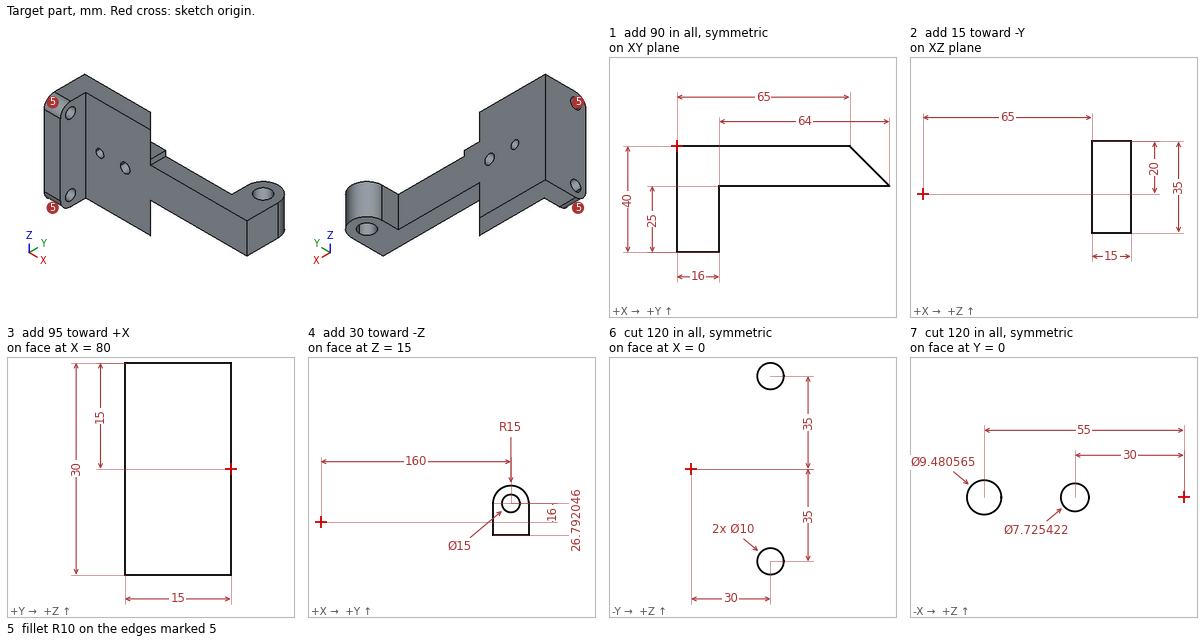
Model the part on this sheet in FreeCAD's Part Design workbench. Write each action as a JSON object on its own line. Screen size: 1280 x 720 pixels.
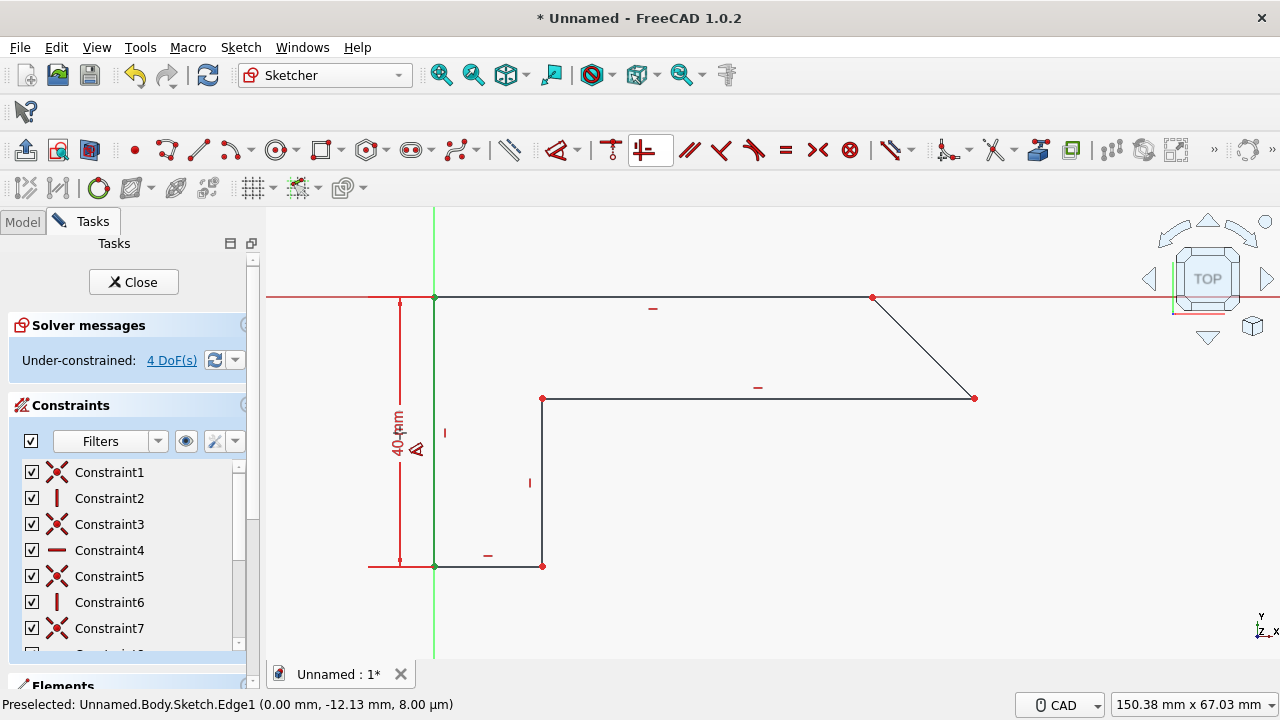
{"action": "left_click", "coordinate": [467, 567]}
{"action": "left_click", "coordinate": [488, 601]}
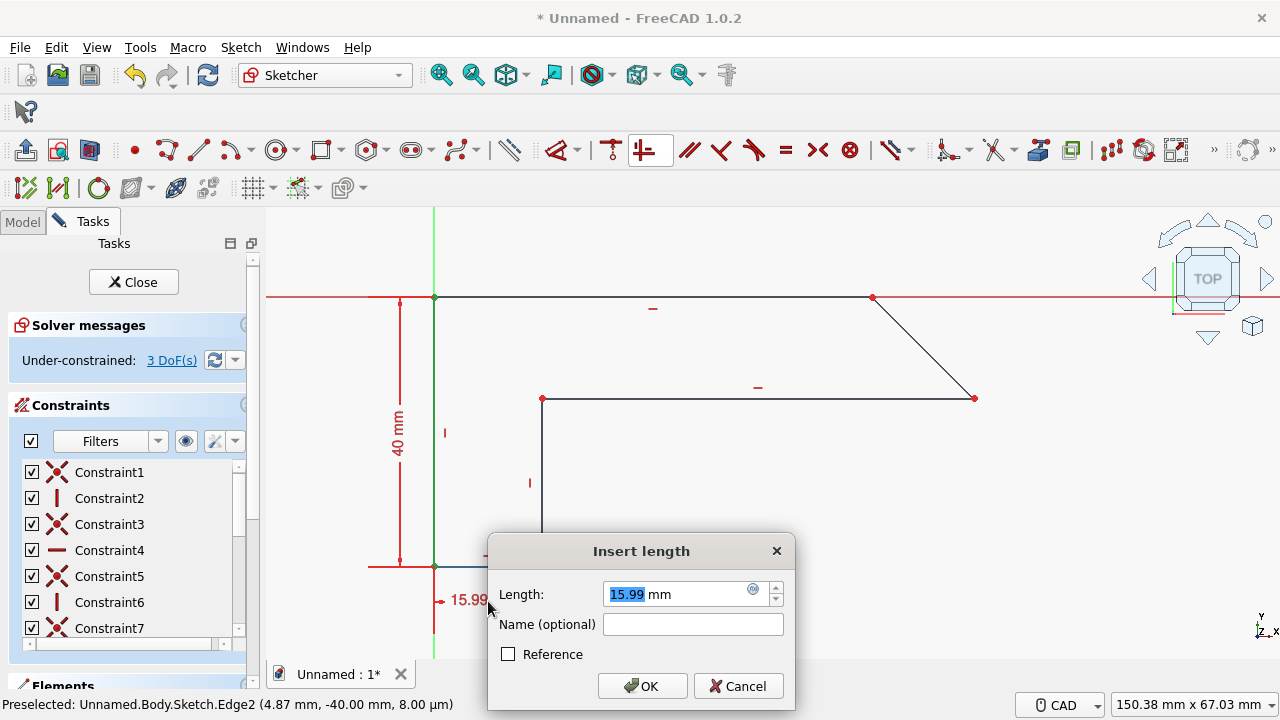
{"action": "type", "text": "16"}
{"action": "key", "text": "Return"}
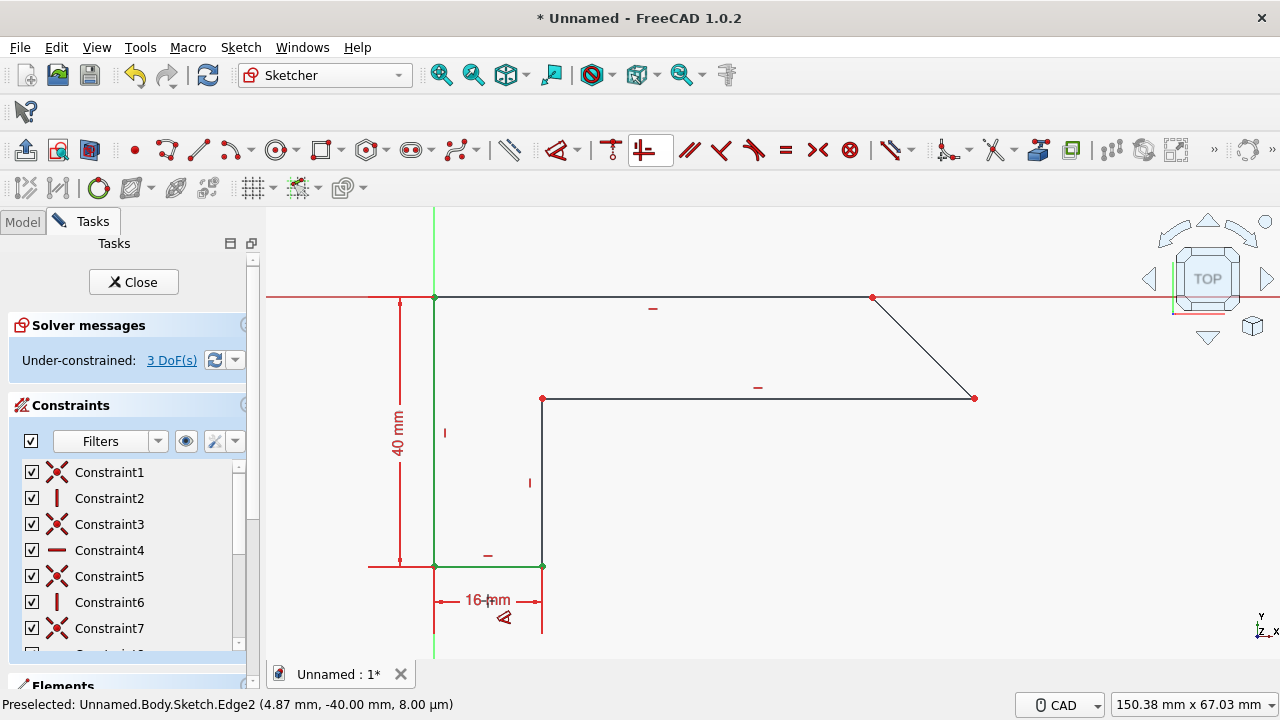
{"action": "left_click", "coordinate": [542, 517]}
{"action": "left_click", "coordinate": [508, 483]}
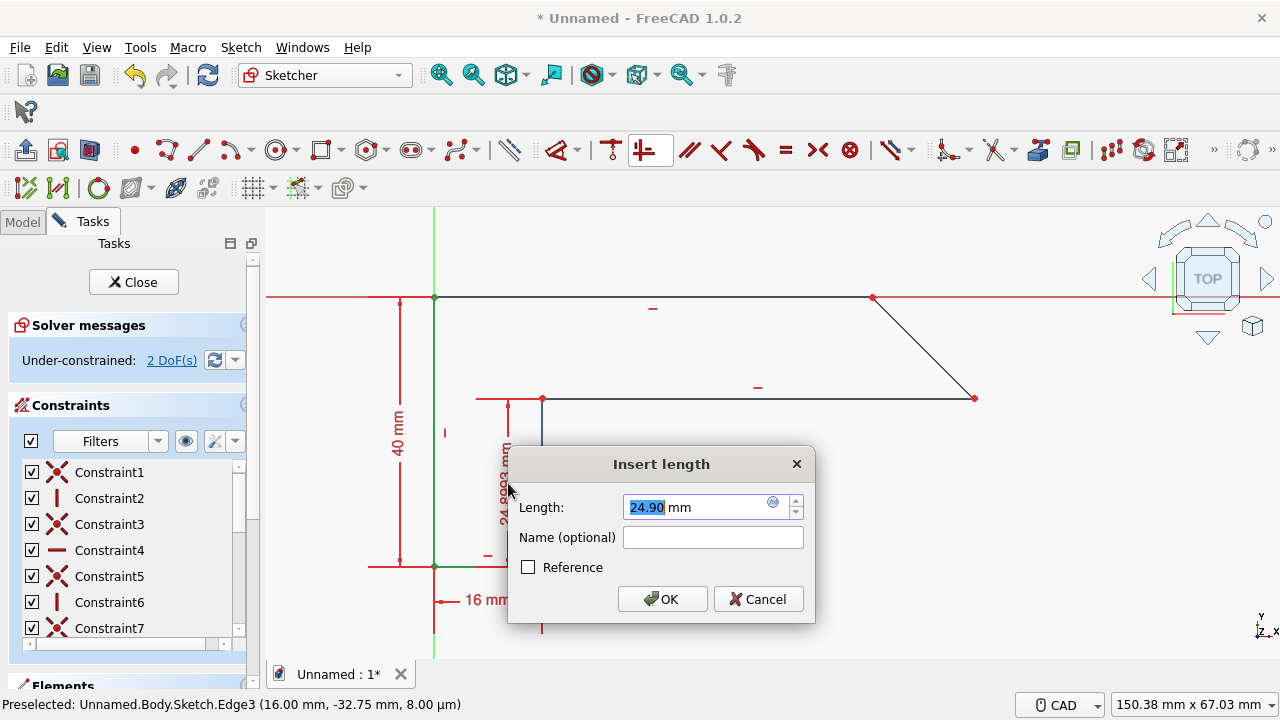
{"action": "type", "text": "25"}
{"action": "key", "text": "Return"}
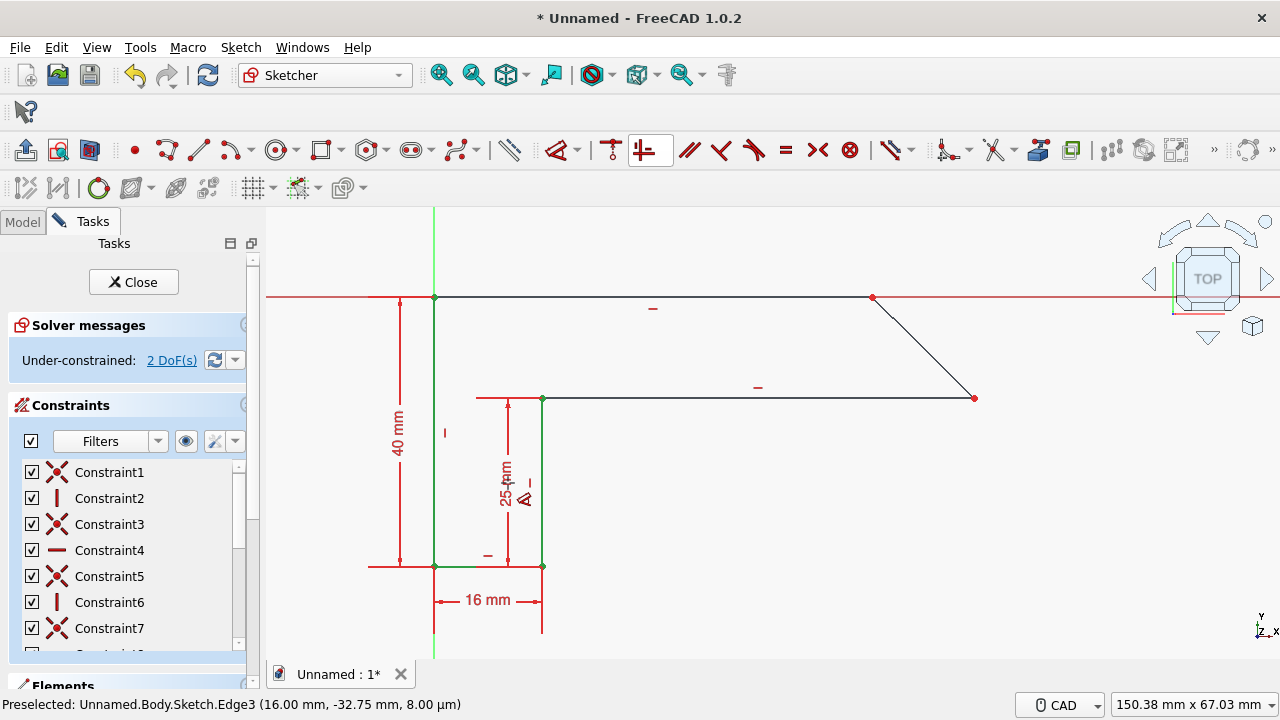
{"action": "left_click", "coordinate": [672, 398]}
{"action": "left_click", "coordinate": [758, 364]}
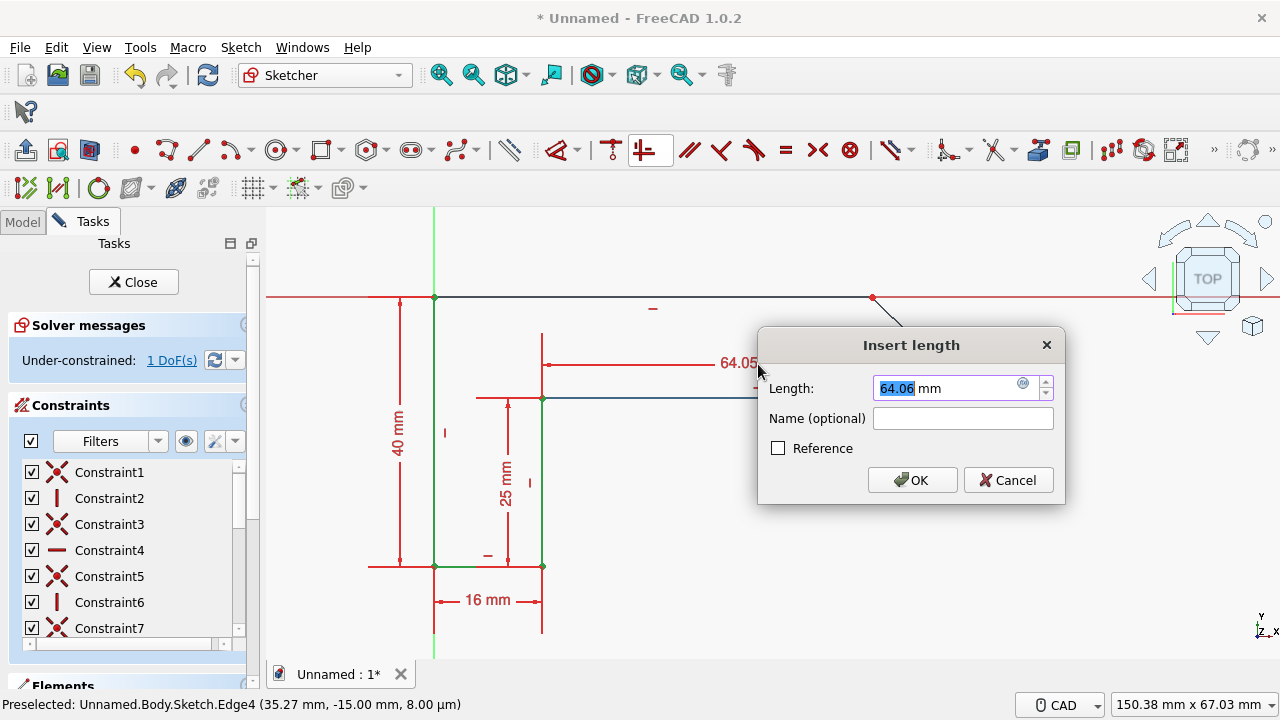
{"action": "type", "text": "64"}
{"action": "key", "text": "Return"}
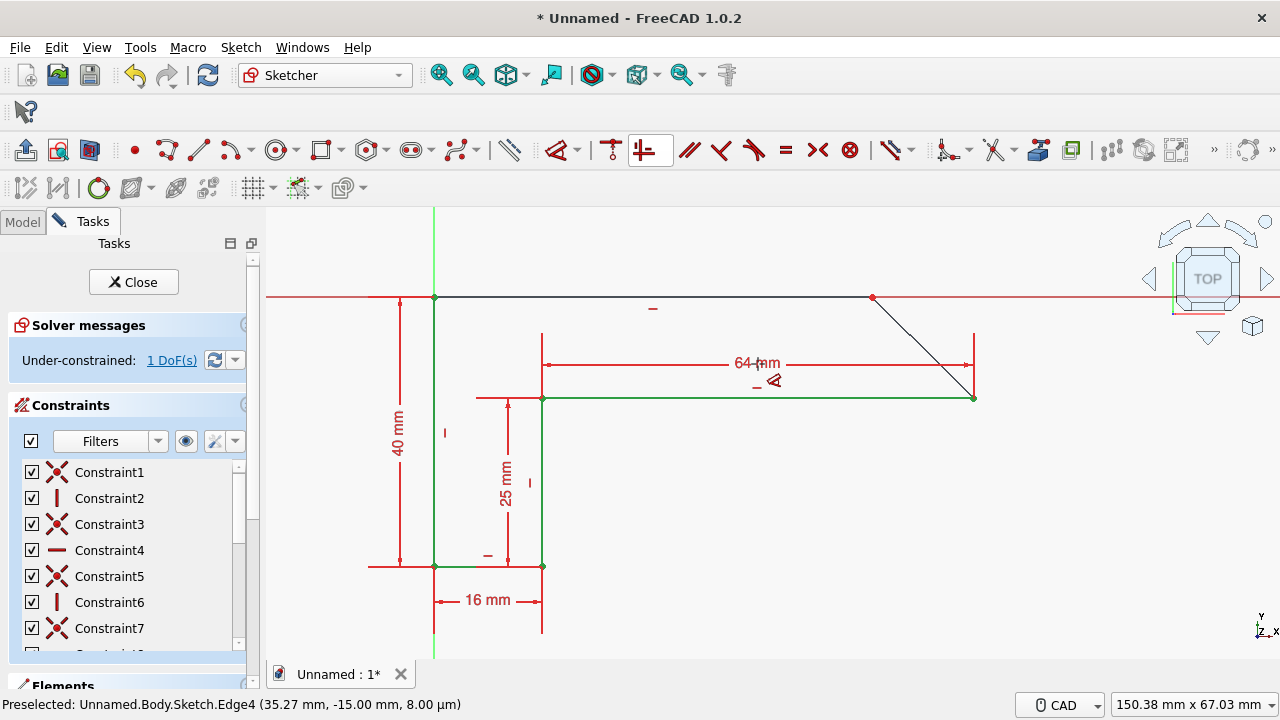
{"action": "left_click", "coordinate": [741, 297]}
{"action": "left_click", "coordinate": [653, 263]}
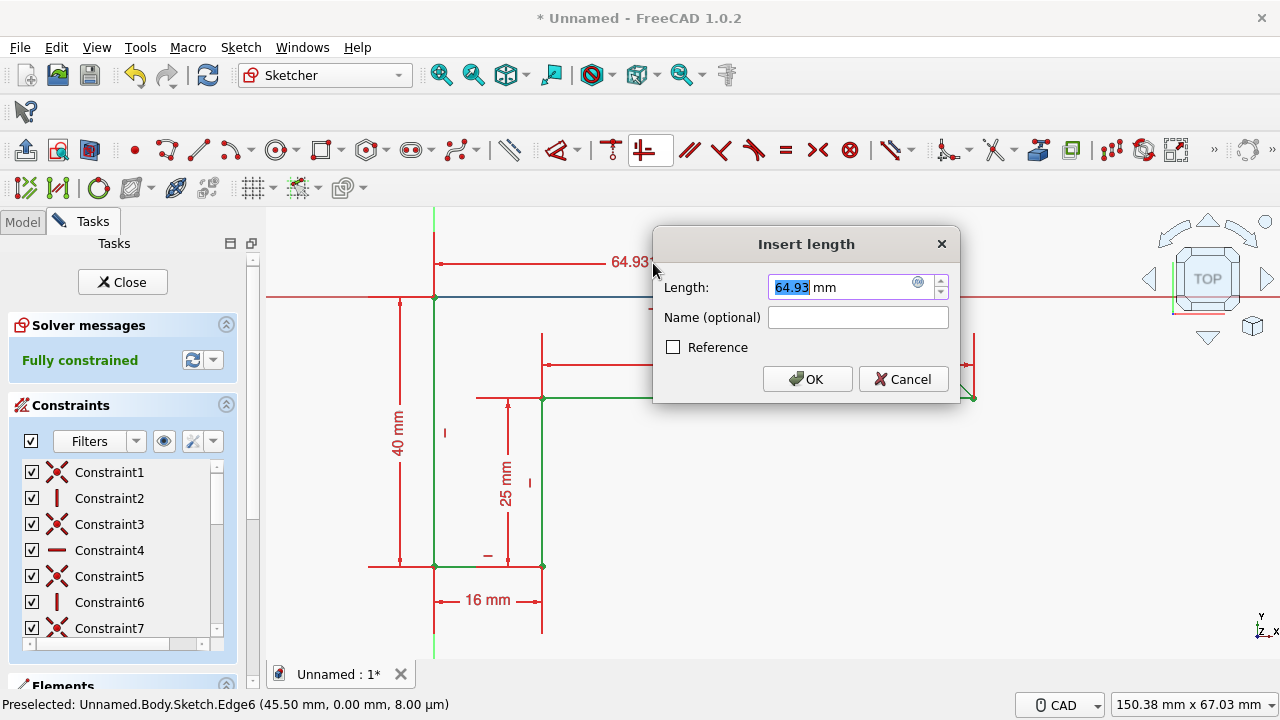
{"action": "type", "text": "65"}
{"action": "key", "text": "Return"}
{"action": "key", "text": "Escape"}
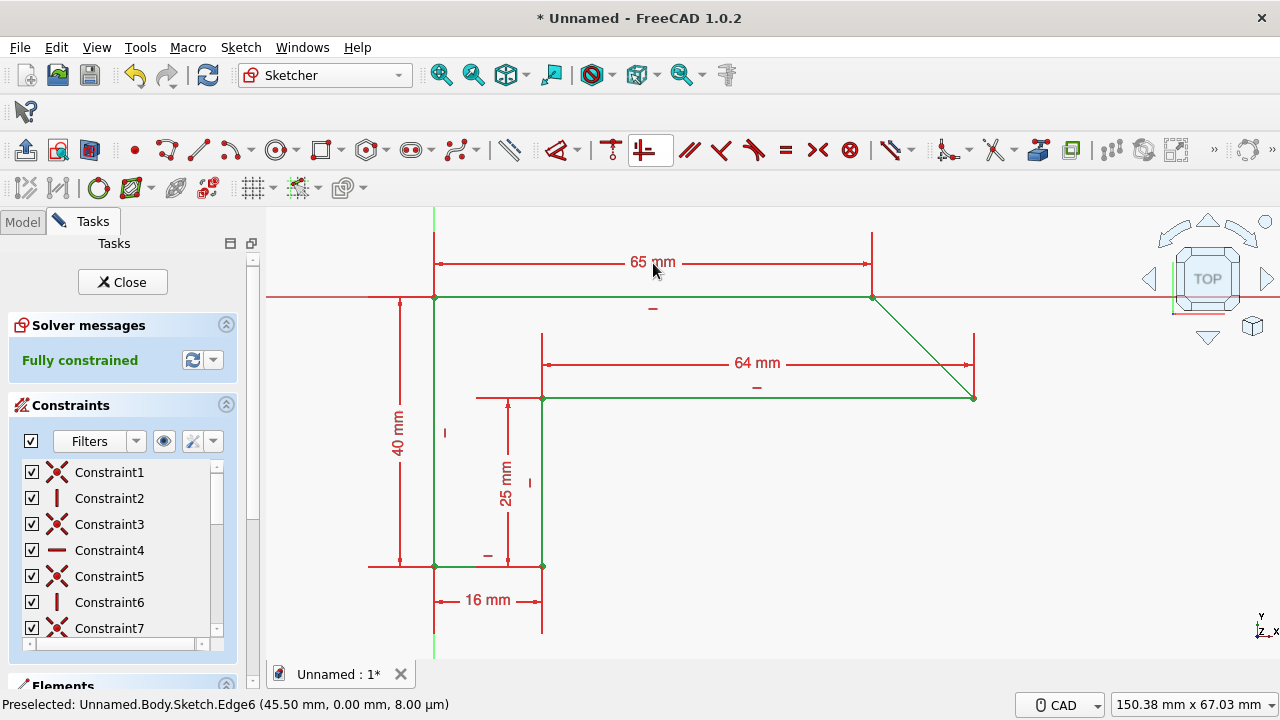
{"action": "left_click", "coordinate": [123, 282]}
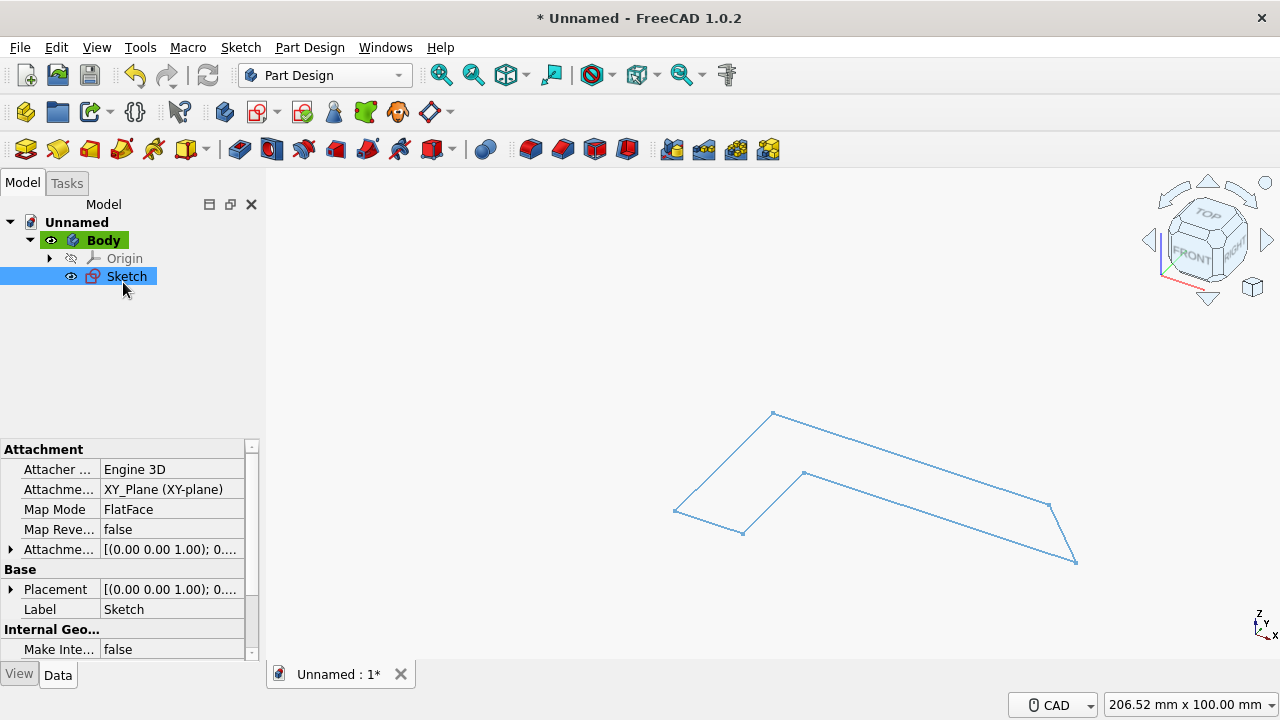
{"action": "left_click", "coordinate": [26, 150]}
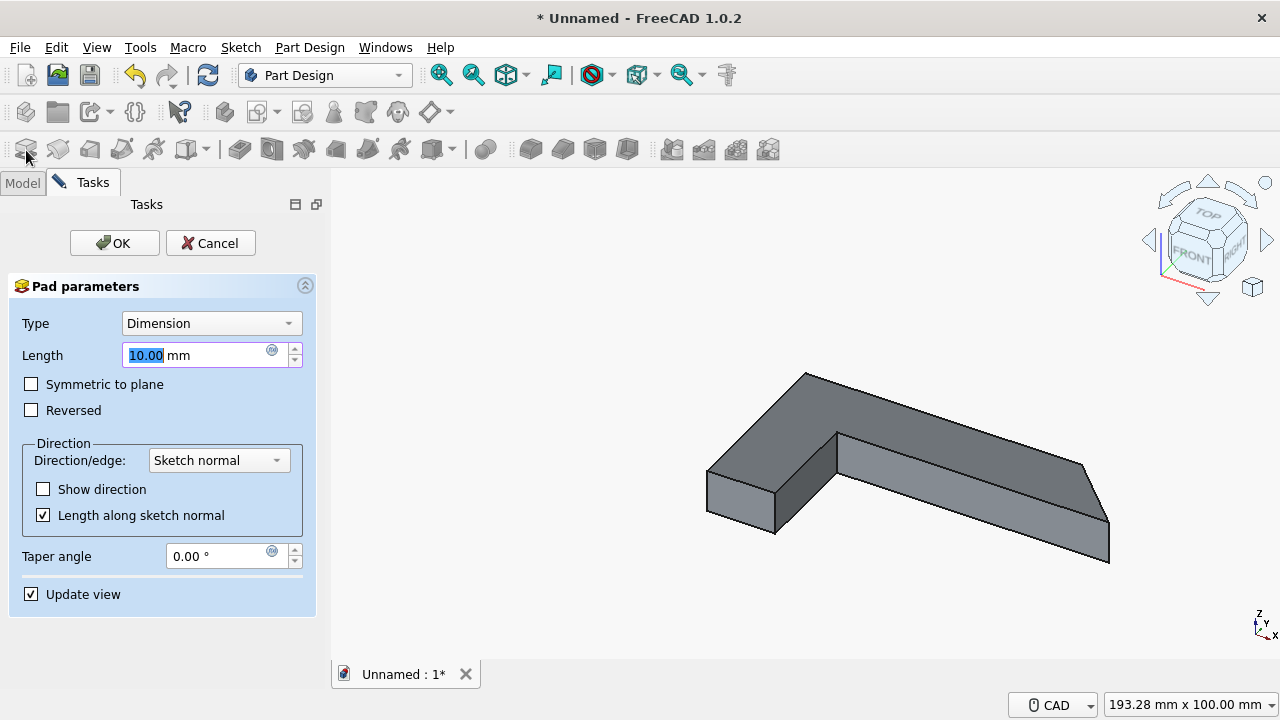
{"action": "type", "text": "90"}
{"action": "key", "text": "Tab"}